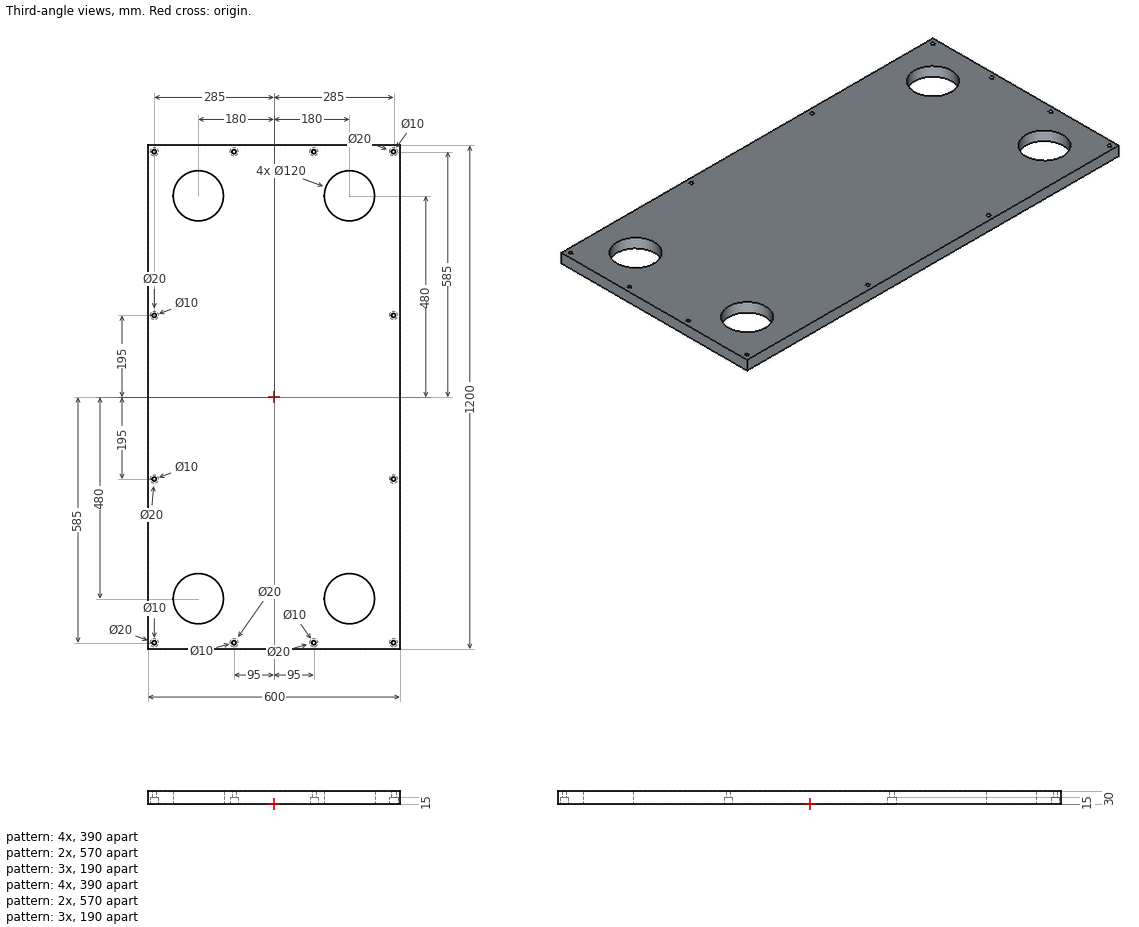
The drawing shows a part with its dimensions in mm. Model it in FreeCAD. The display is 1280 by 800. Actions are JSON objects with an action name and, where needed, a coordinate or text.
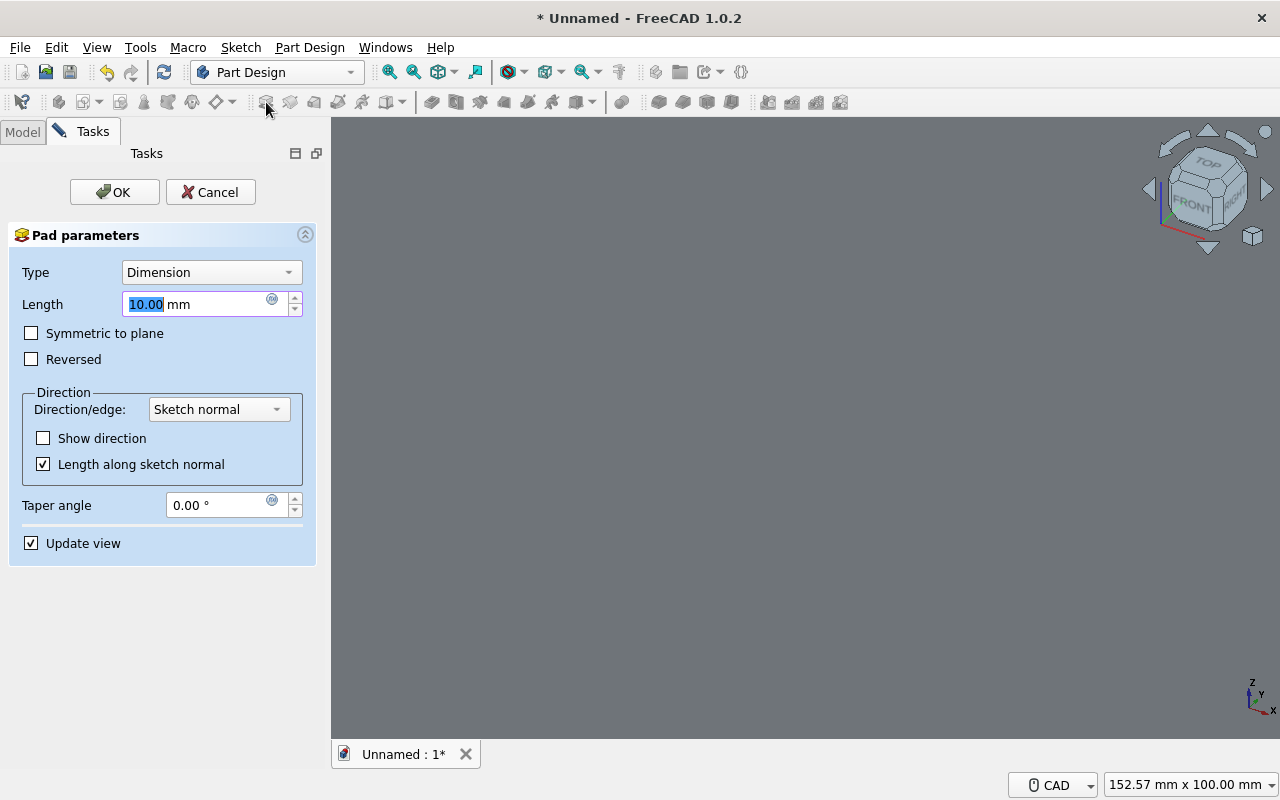
{"action": "type", "text": "30"}
{"action": "key", "text": "Tab"}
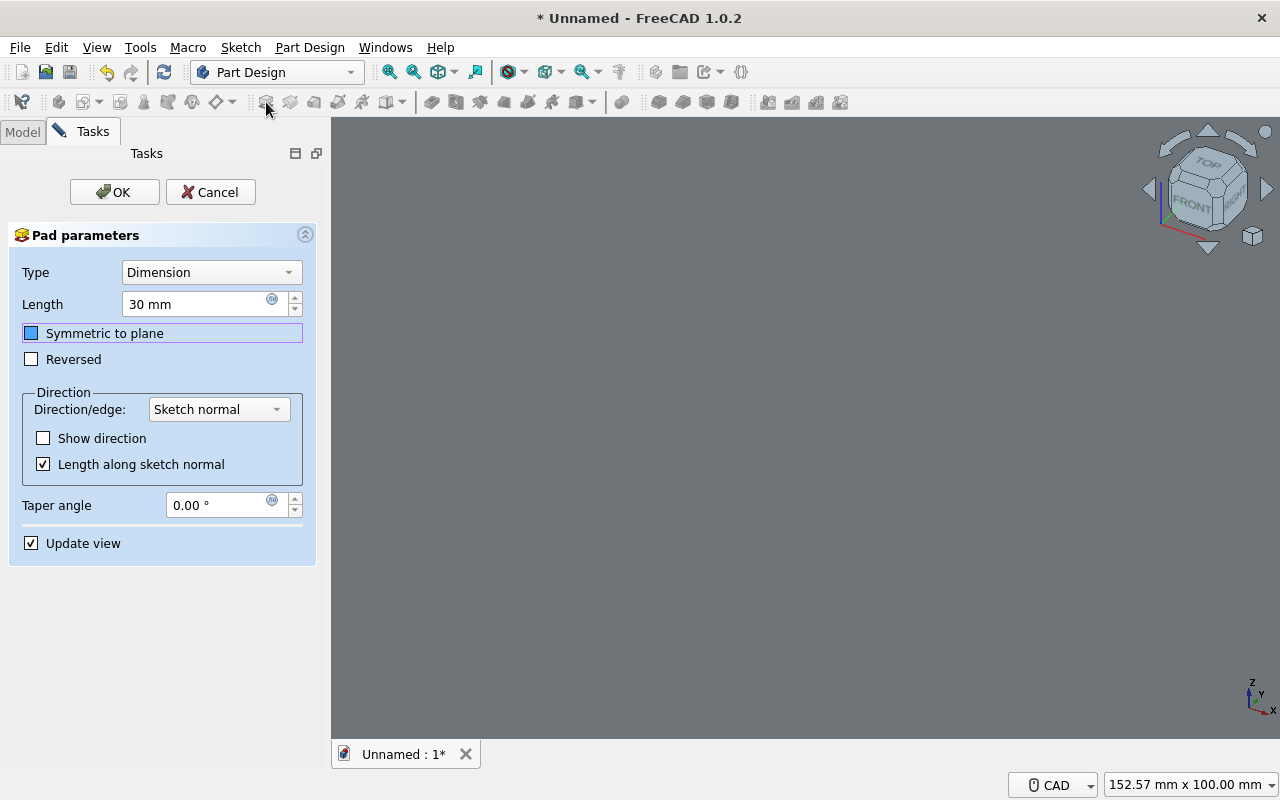
{"action": "left_click", "coordinate": [115, 192]}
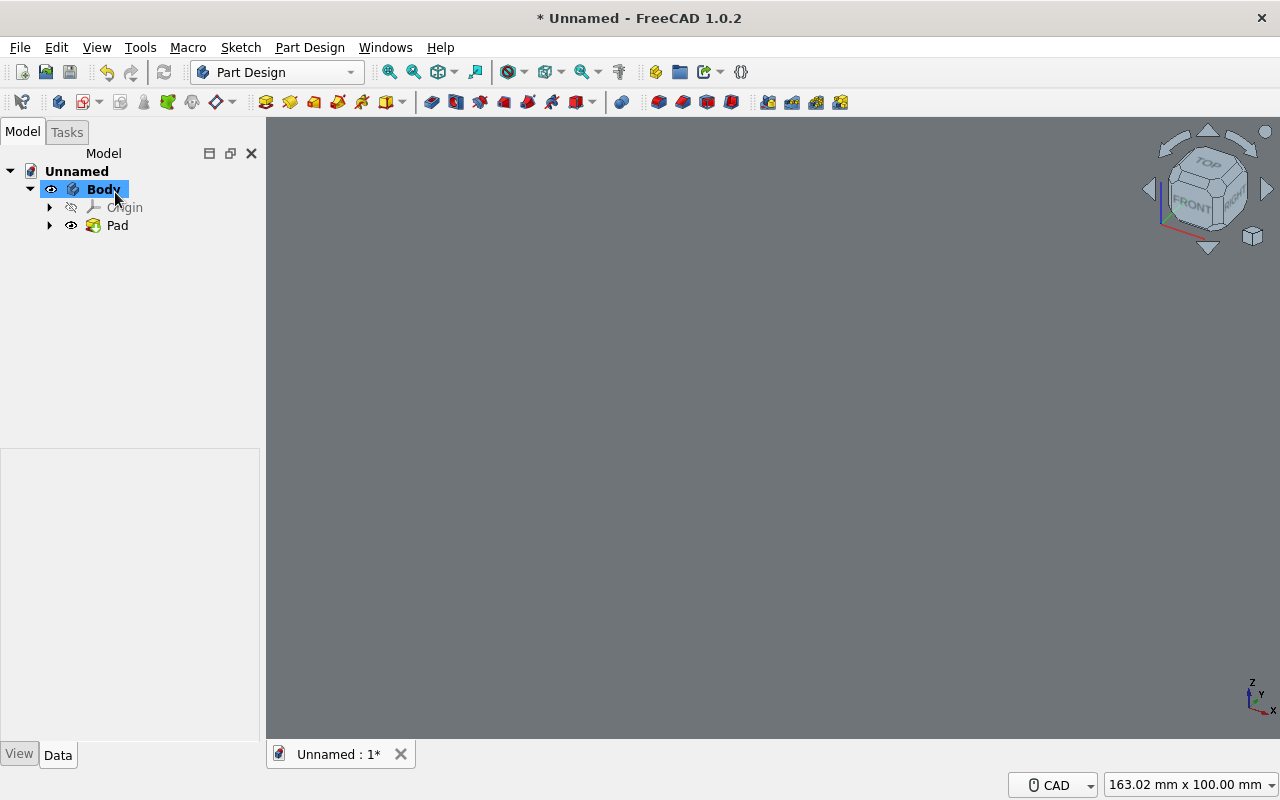
{"action": "left_click", "coordinate": [390, 72]}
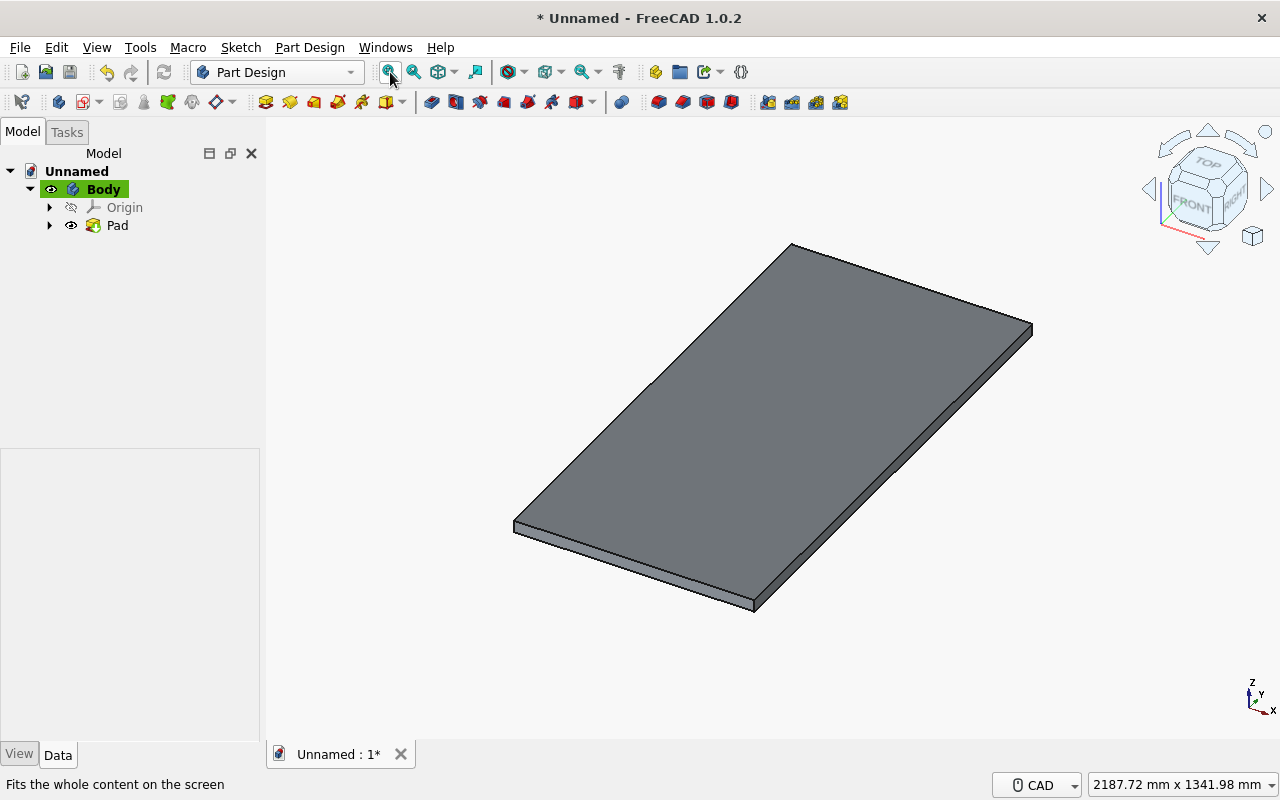
{"action": "key", "text": "5"}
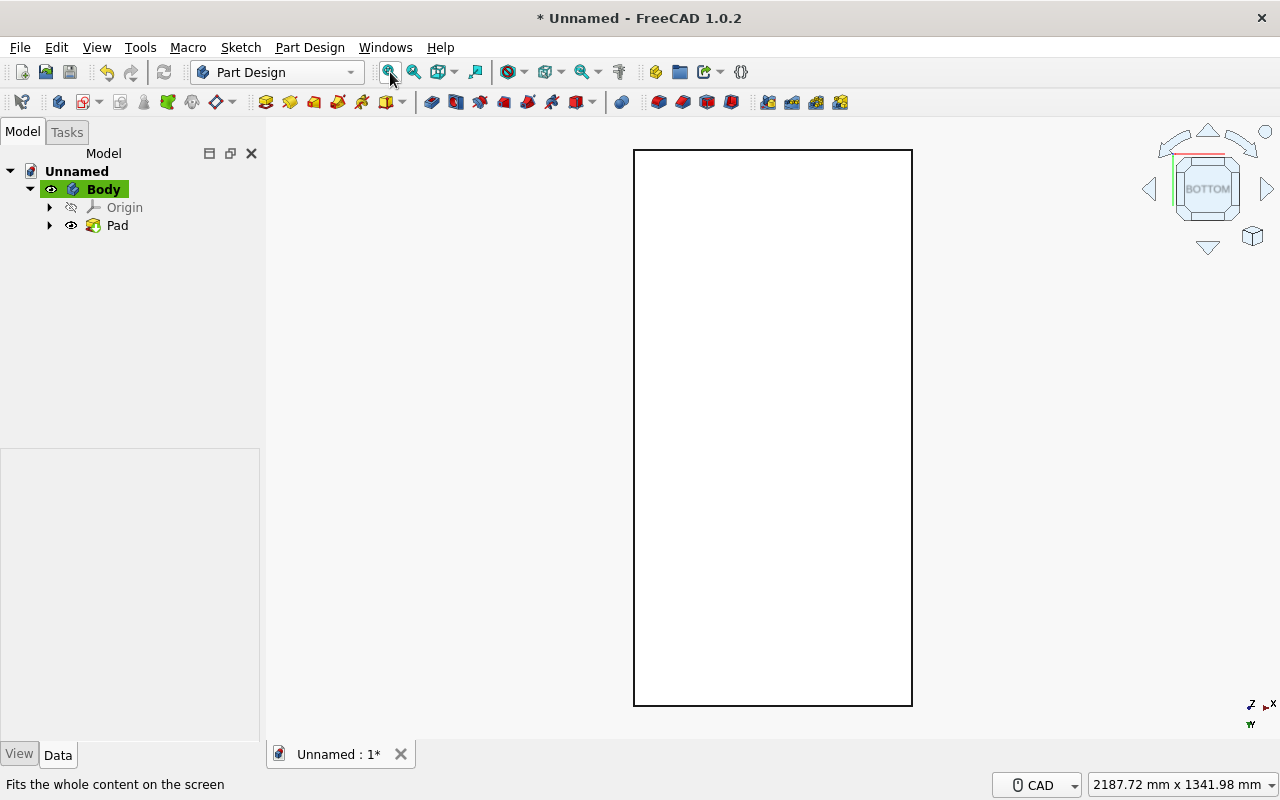
{"action": "left_click", "coordinate": [773, 506]}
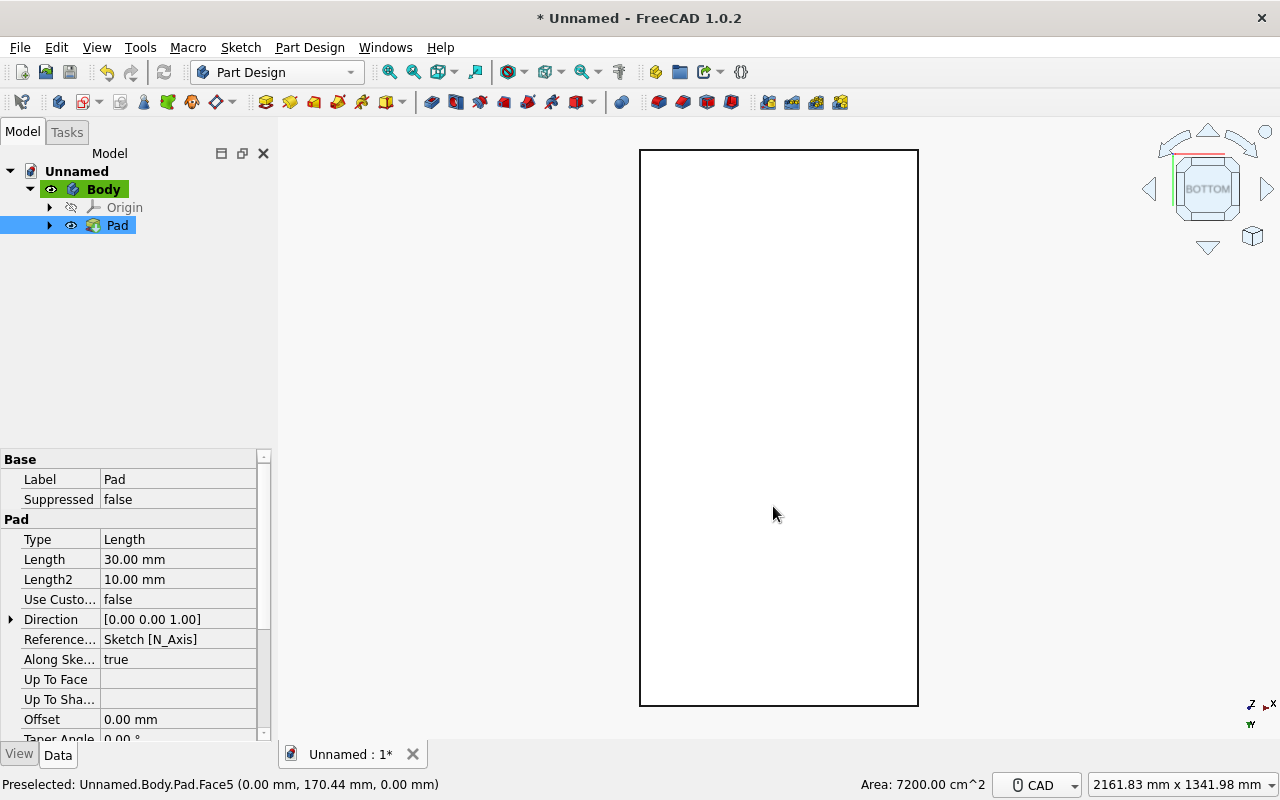
{"action": "left_click", "coordinate": [84, 102]}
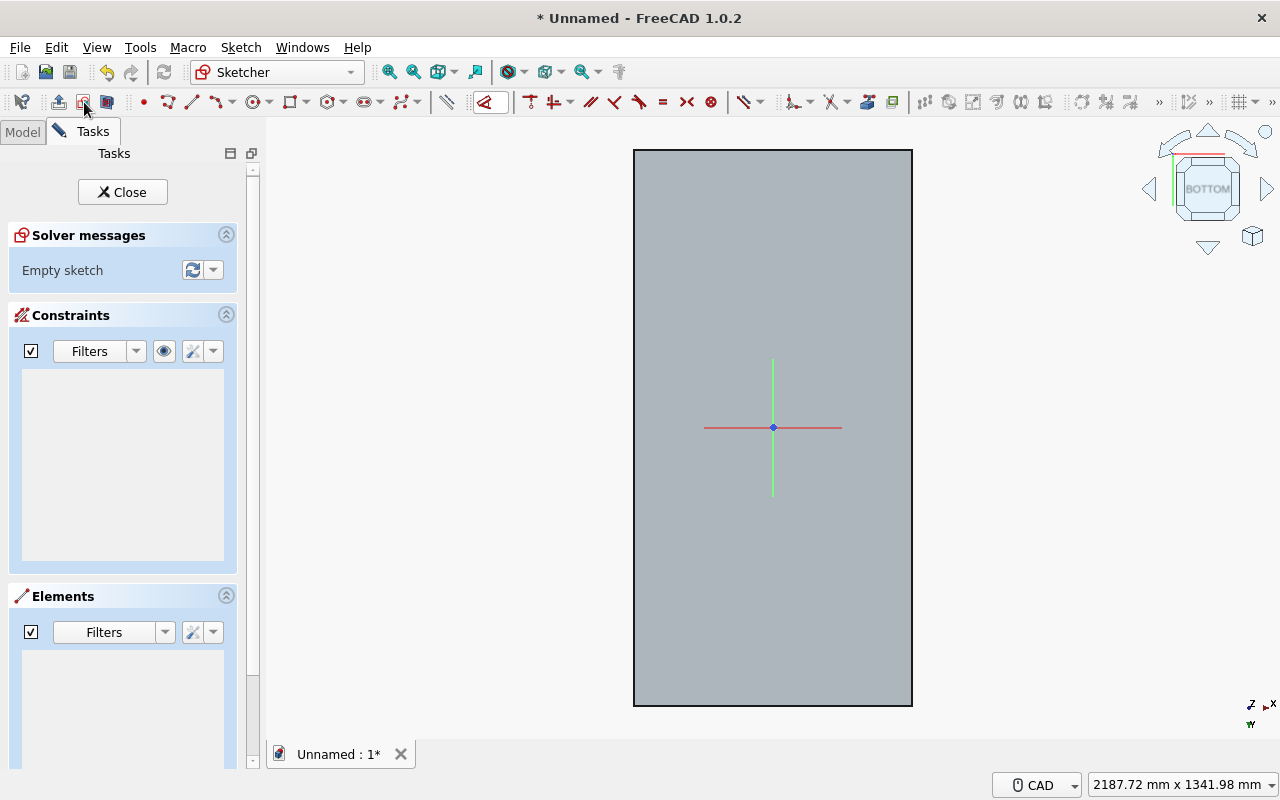
{"action": "left_click", "coordinate": [254, 102]}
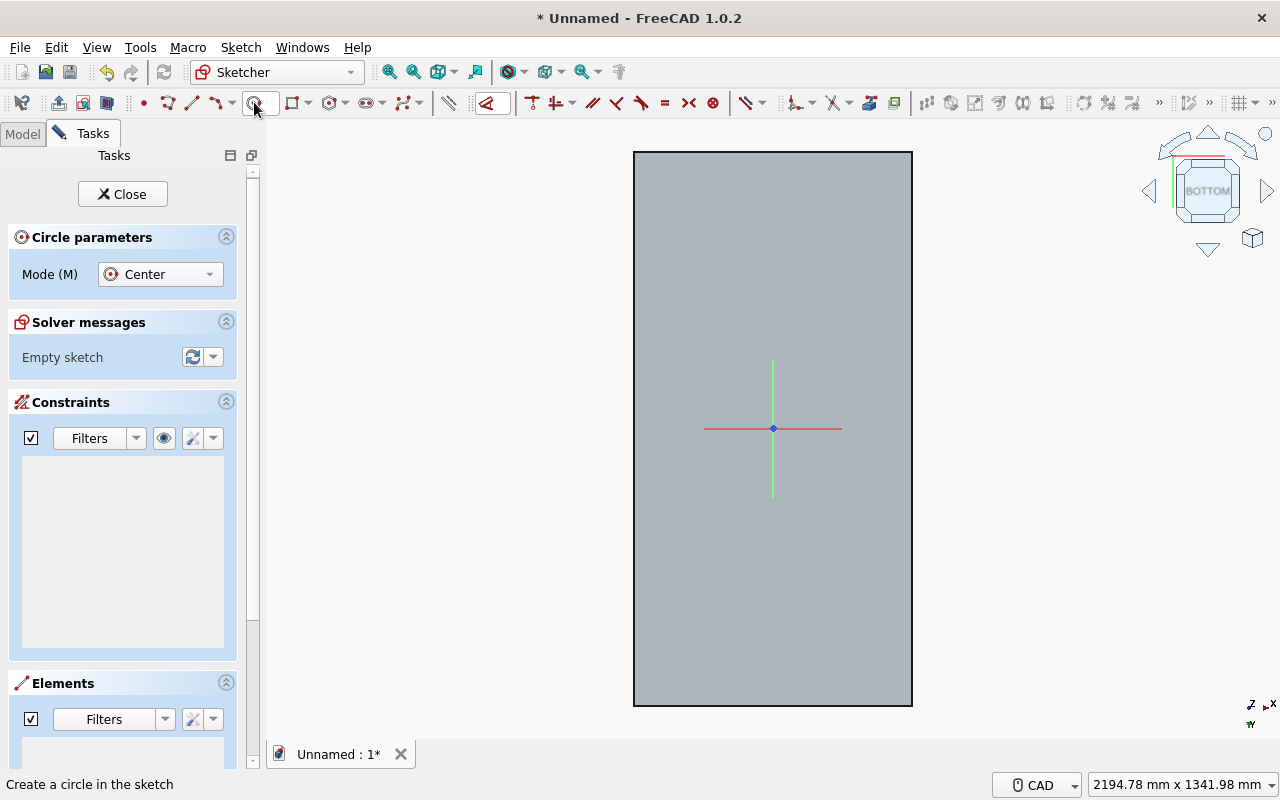
{"action": "left_click", "coordinate": [856, 651]}
{"action": "mouse_move", "coordinate": [876, 631]}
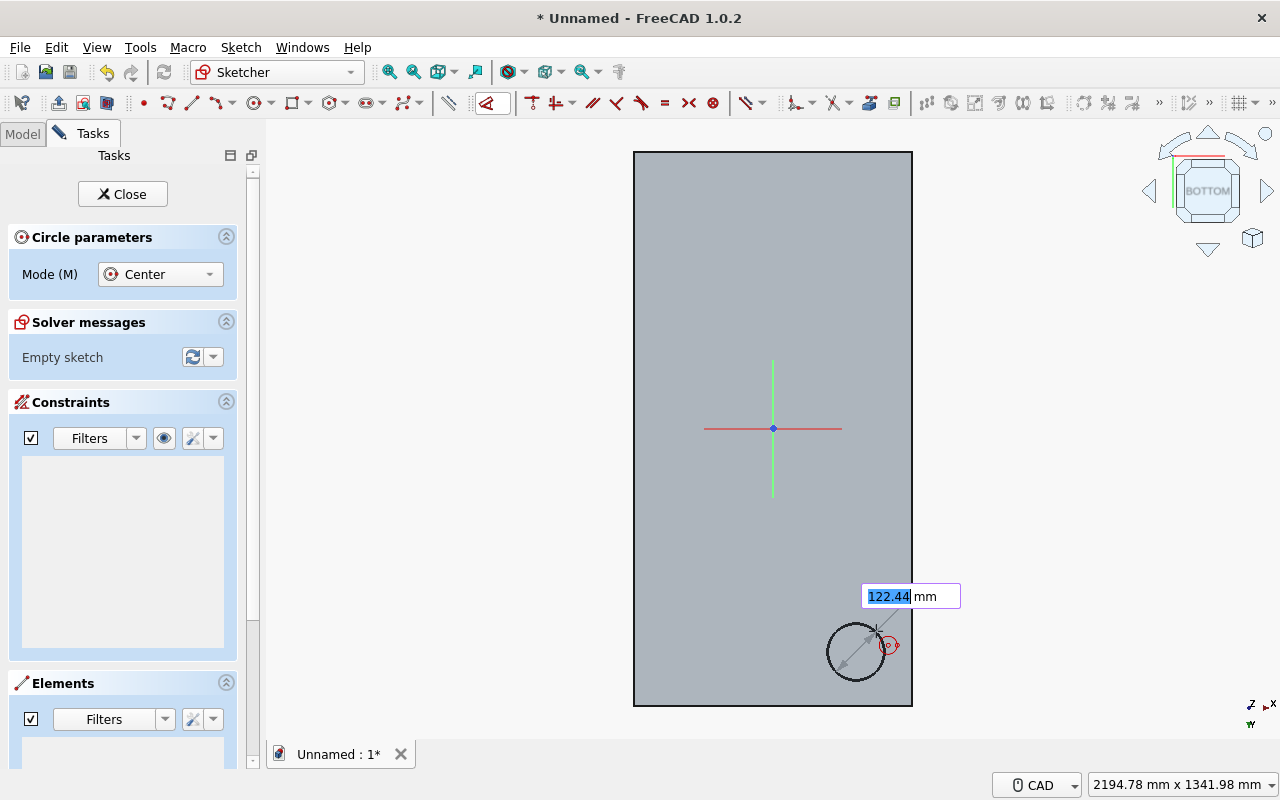
{"action": "type", "text": "120"}
{"action": "key", "text": "Return"}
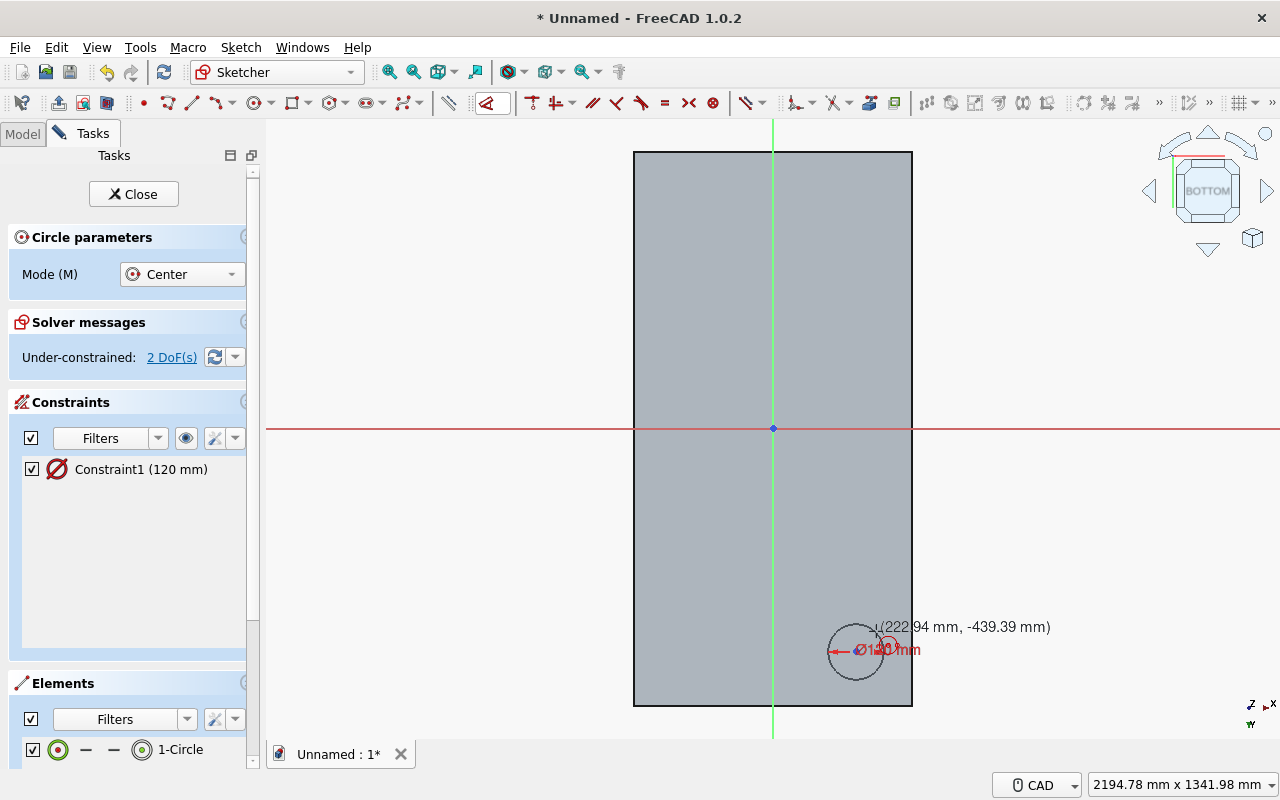
{"action": "left_click", "coordinate": [690, 651]}
{"action": "mouse_move", "coordinate": [709, 631]}